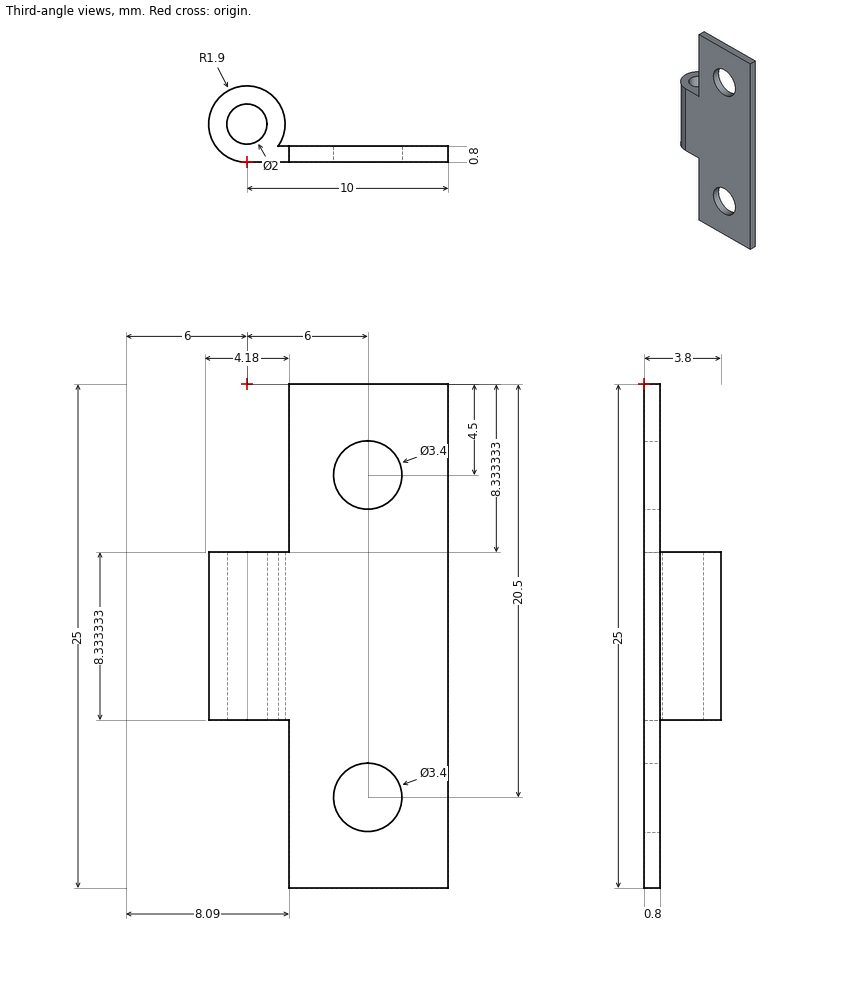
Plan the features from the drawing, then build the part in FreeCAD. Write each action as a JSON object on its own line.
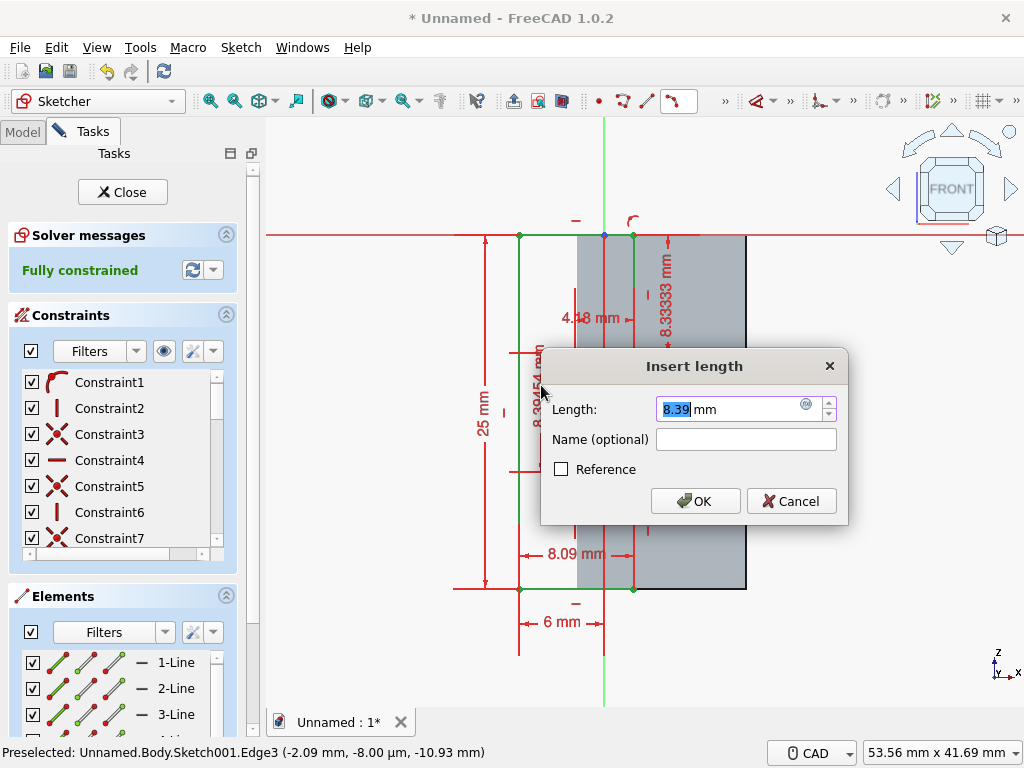
{"action": "type", "text": "8.333333"}
{"action": "key", "text": "Return"}
{"action": "key", "text": "Escape"}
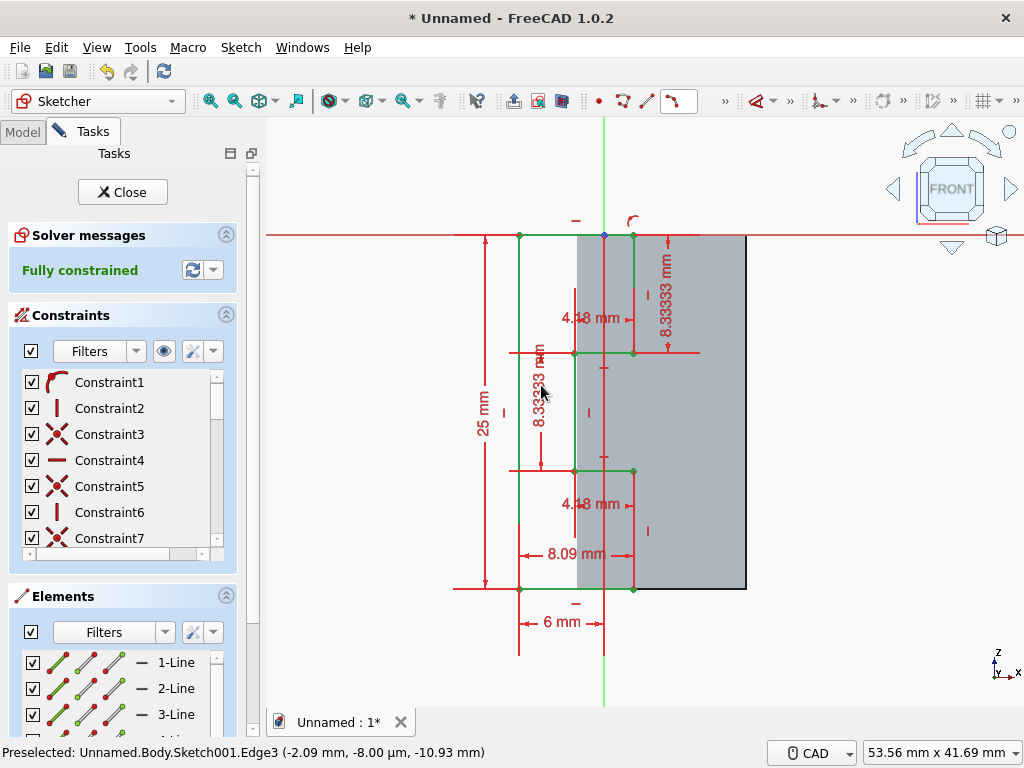
{"action": "left_click", "coordinate": [123, 192]}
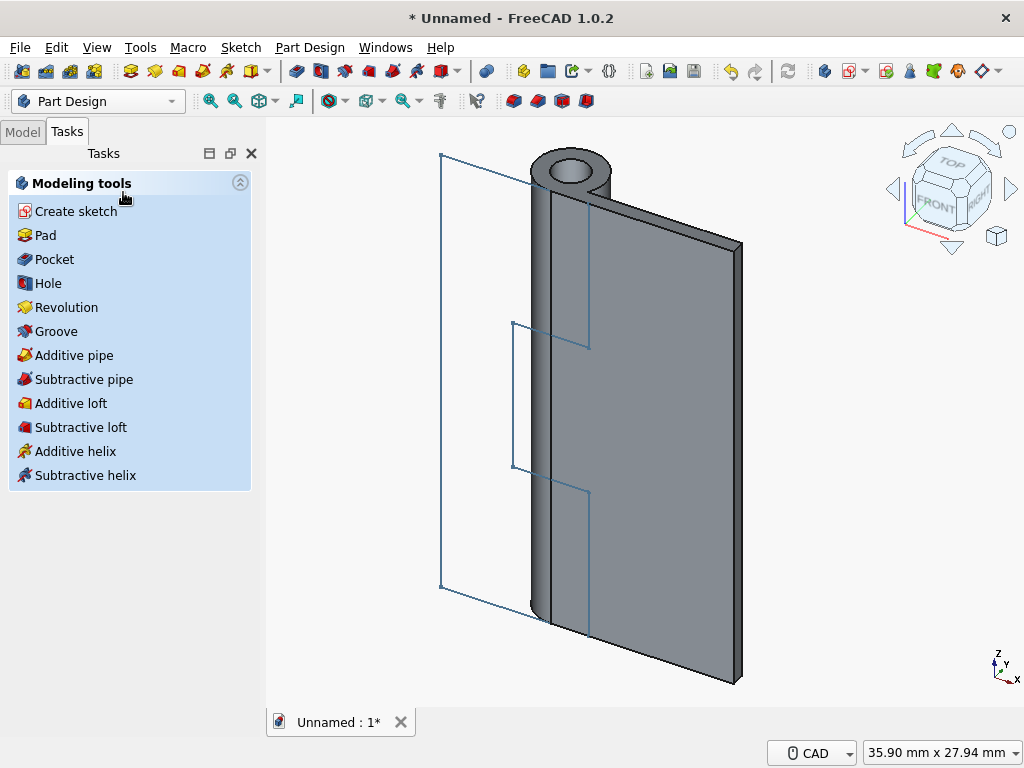
{"action": "left_click", "coordinate": [298, 72]}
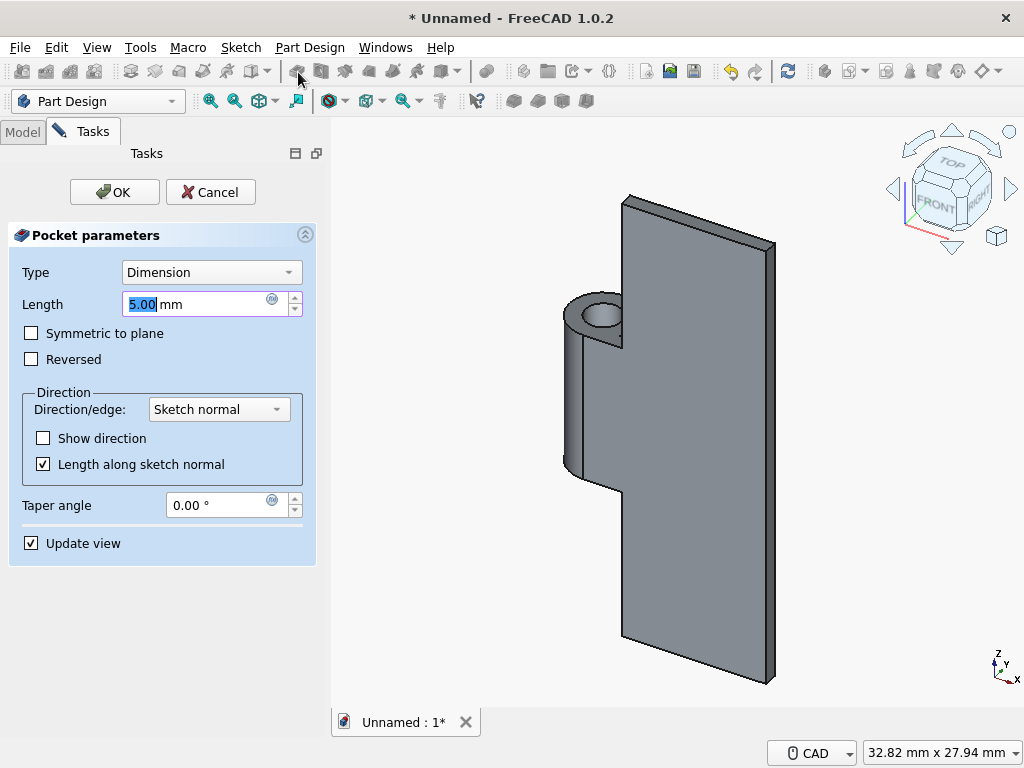
{"action": "type", "text": "3.8"}
{"action": "key", "text": "Tab"}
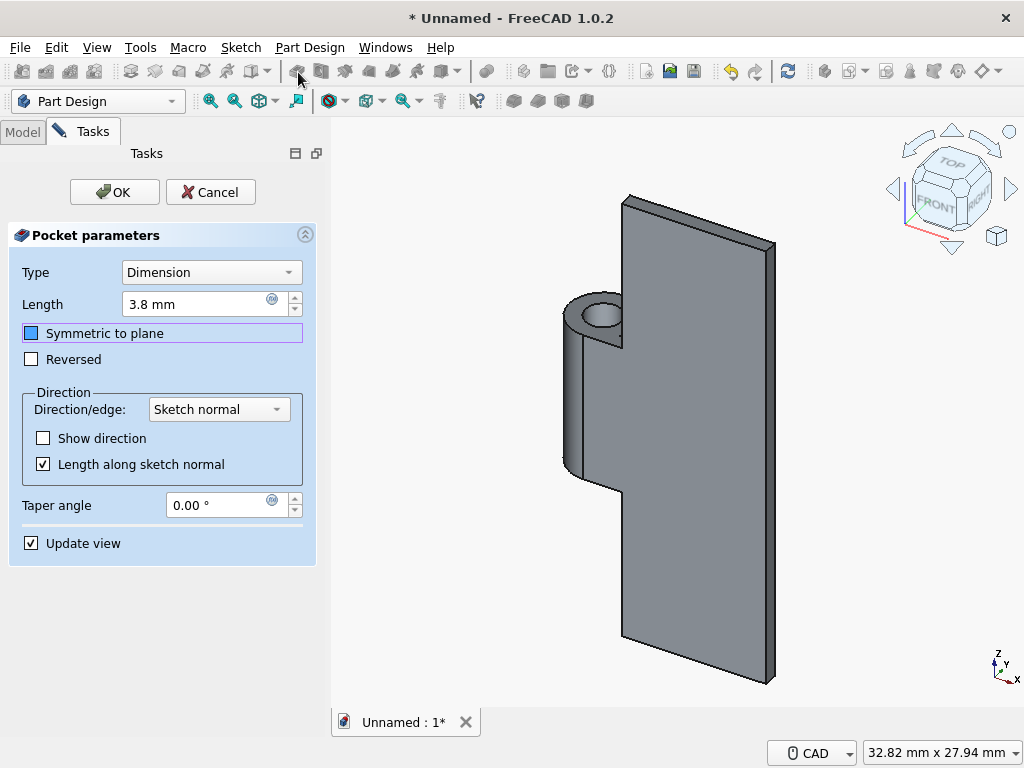
{"action": "left_click", "coordinate": [115, 192]}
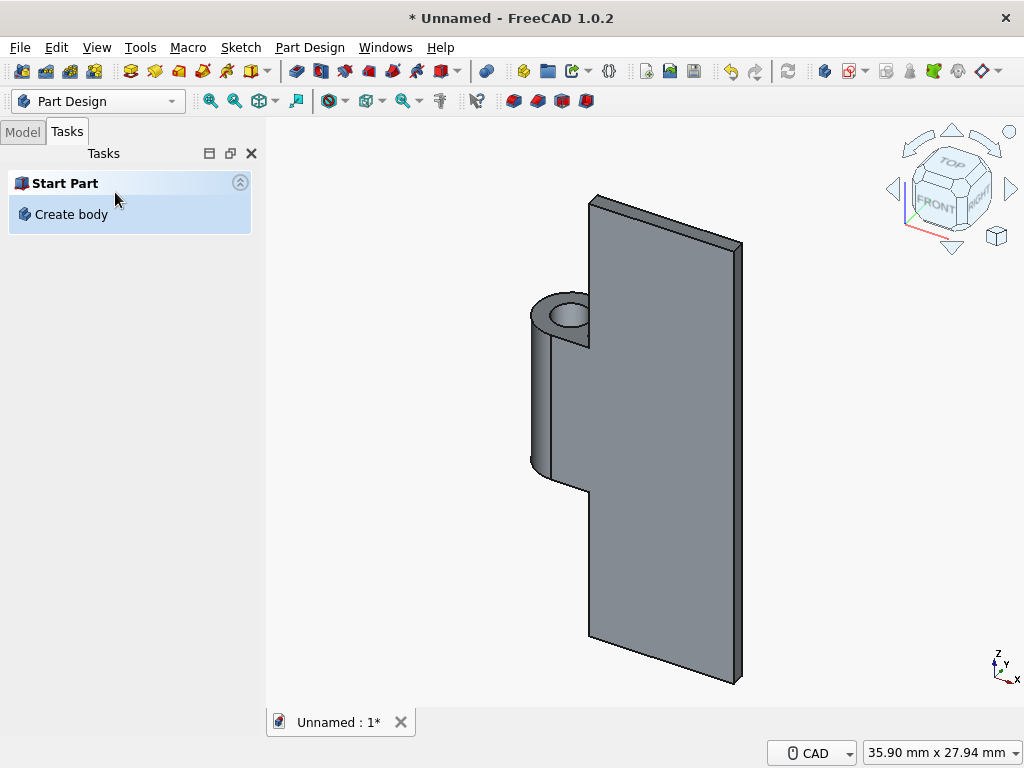
{"action": "left_click", "coordinate": [850, 72]}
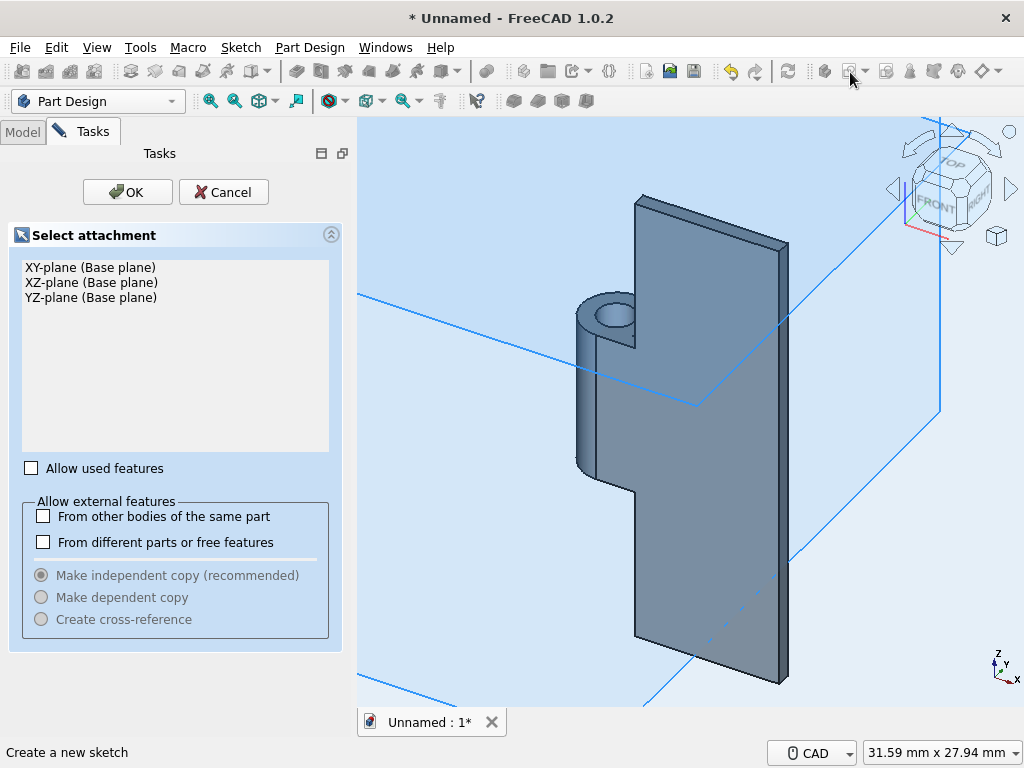
{"action": "left_click", "coordinate": [82, 282]}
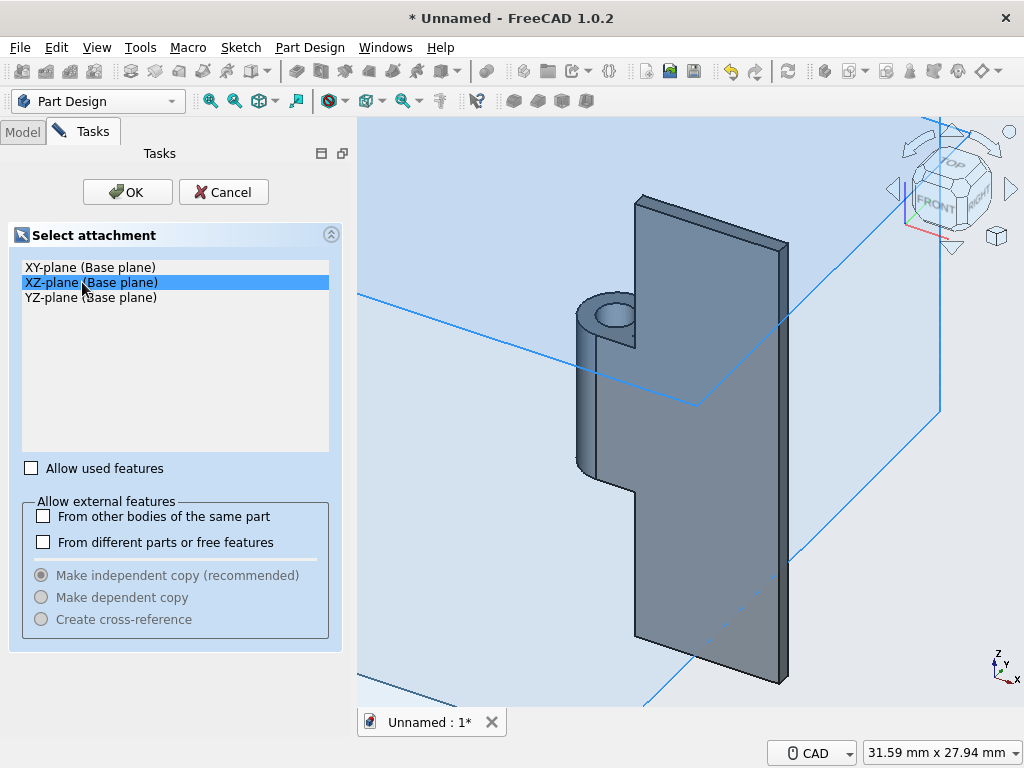
{"action": "left_click", "coordinate": [128, 192]}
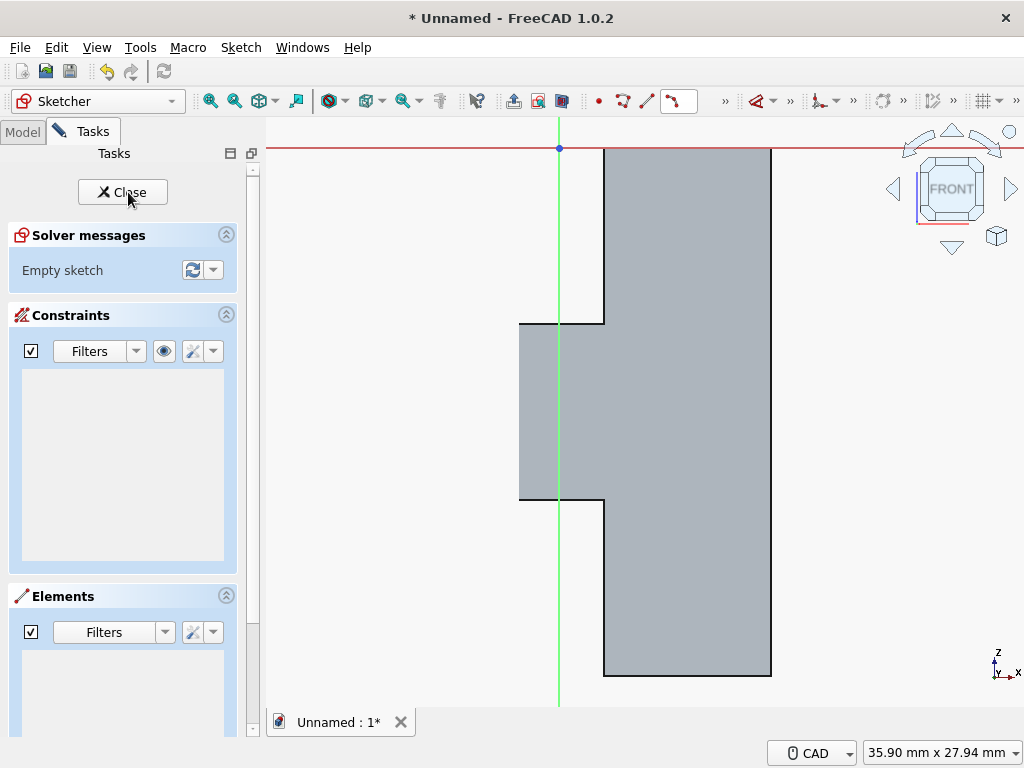
{"action": "scroll", "coordinate": [714, 624], "scroll_direction": "up", "scroll_amount": 8}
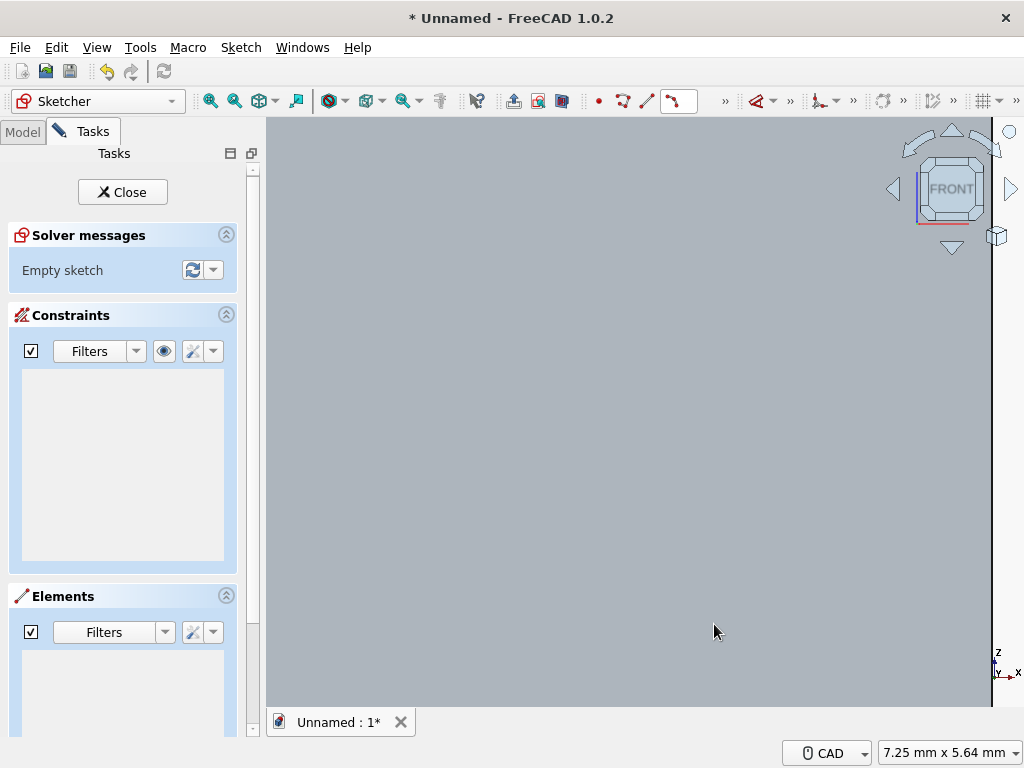
{"action": "key", "text": "g c"}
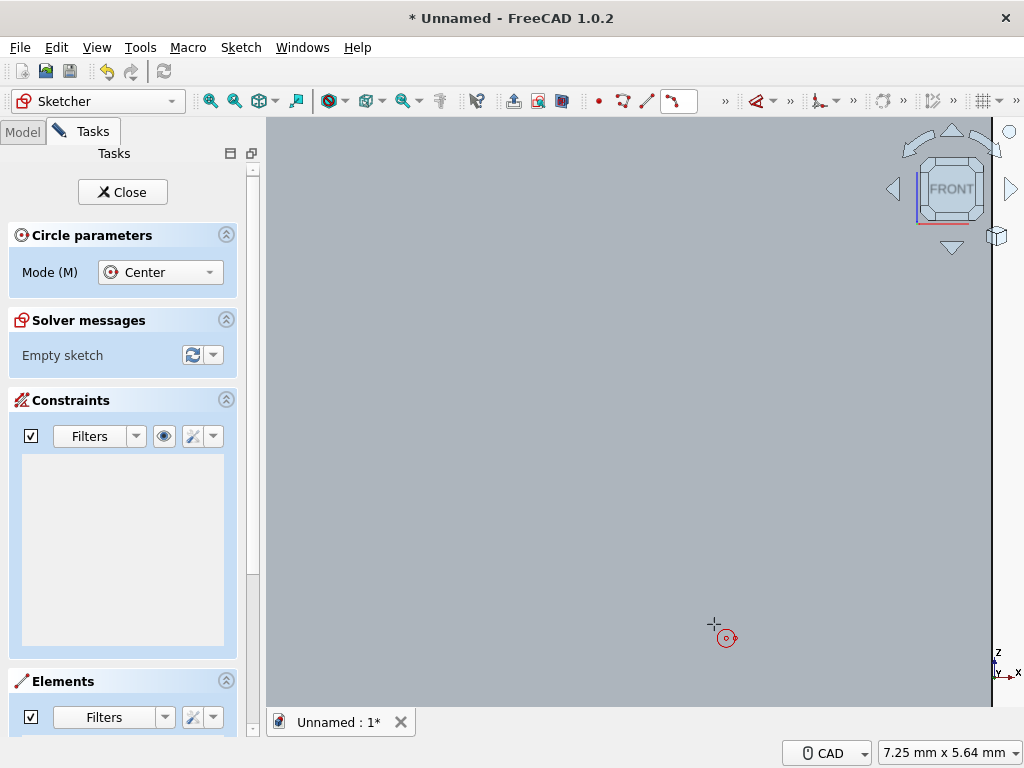
{"action": "left_click", "coordinate": [574, 407]}
{"action": "left_click", "coordinate": [699, 281]}
{"action": "key", "text": "Escape"}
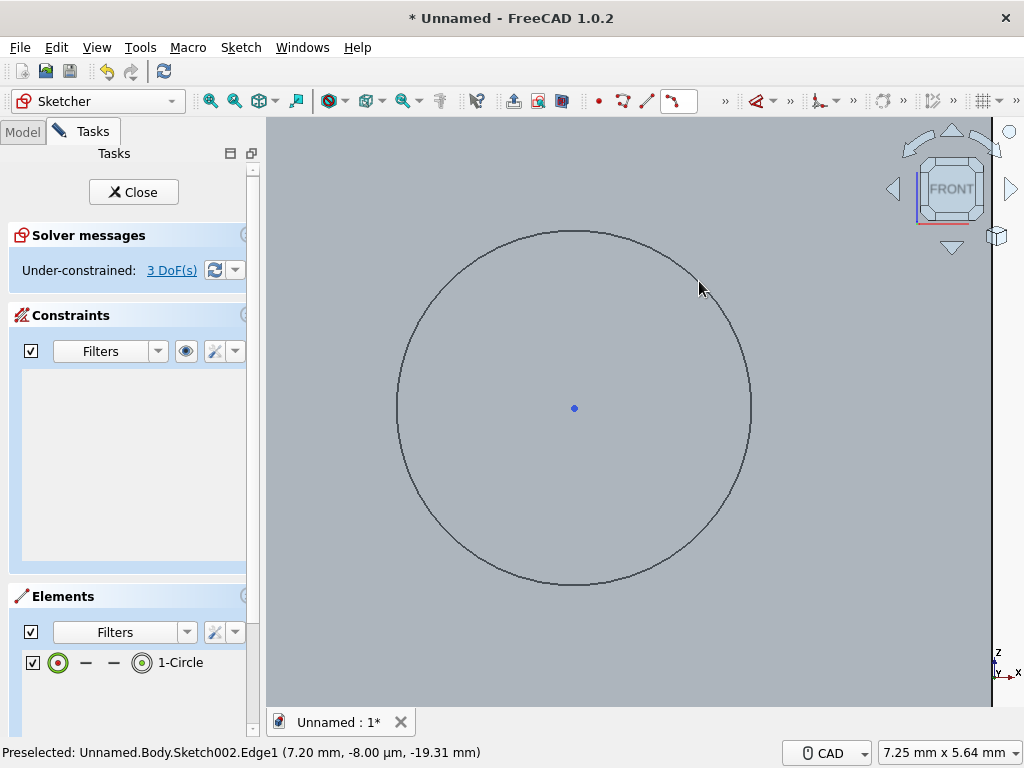
{"action": "left_click", "coordinate": [756, 102]}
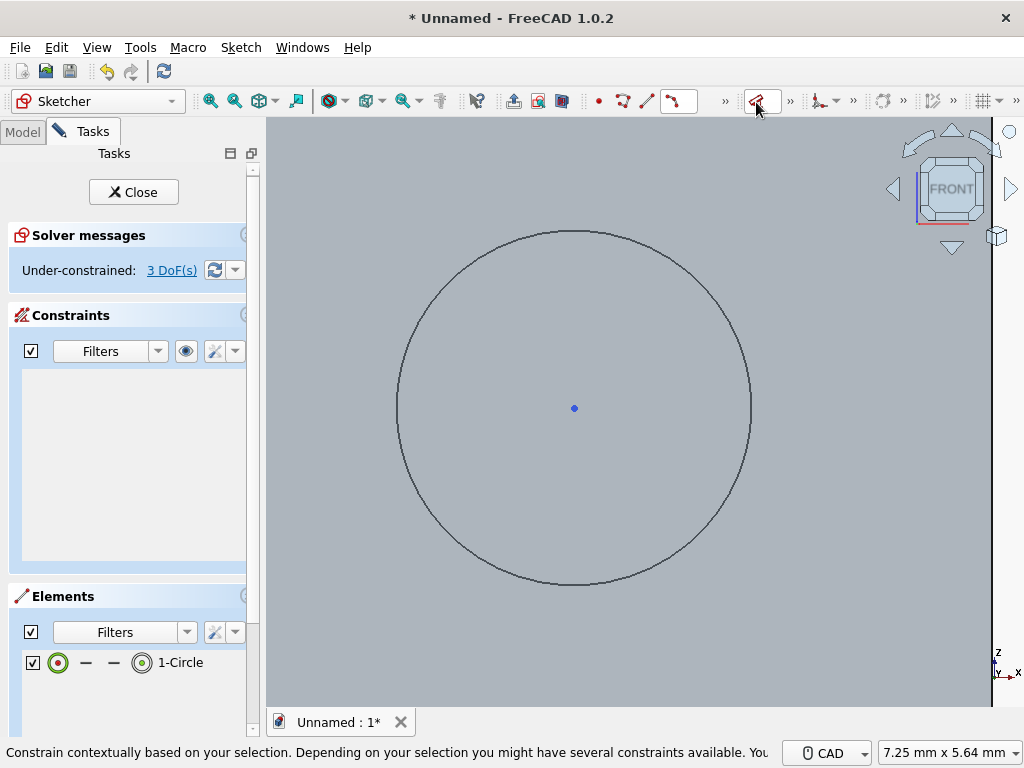
{"action": "left_click", "coordinate": [699, 282]}
{"action": "left_click", "coordinate": [722, 259]}